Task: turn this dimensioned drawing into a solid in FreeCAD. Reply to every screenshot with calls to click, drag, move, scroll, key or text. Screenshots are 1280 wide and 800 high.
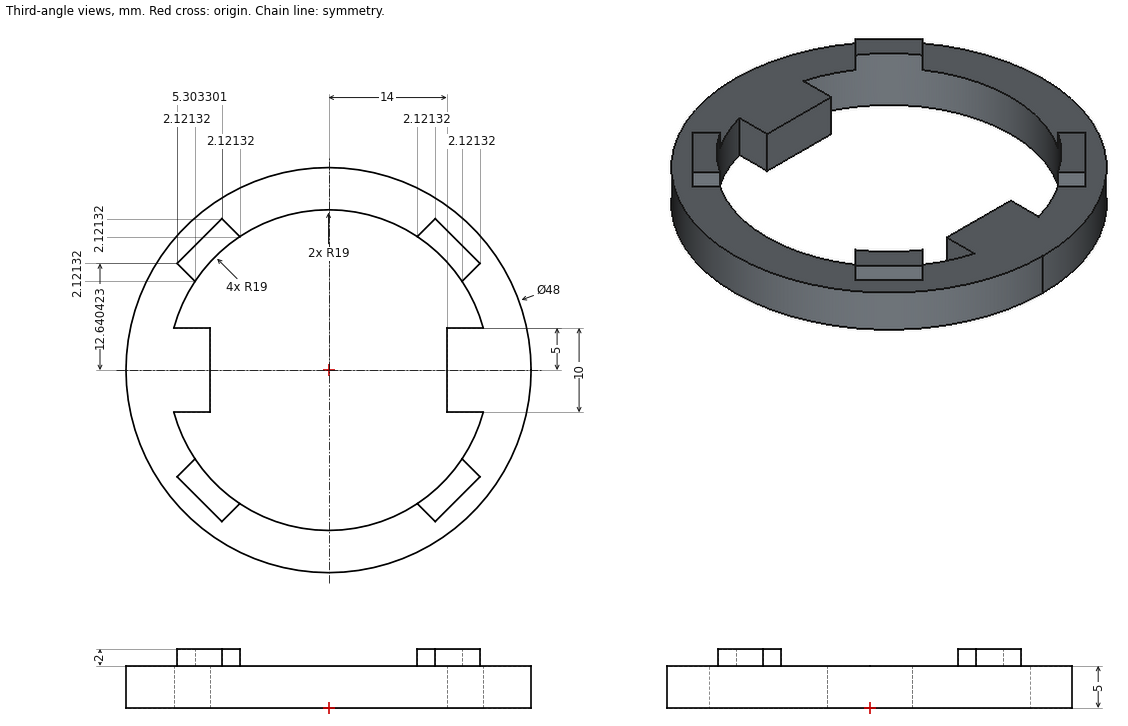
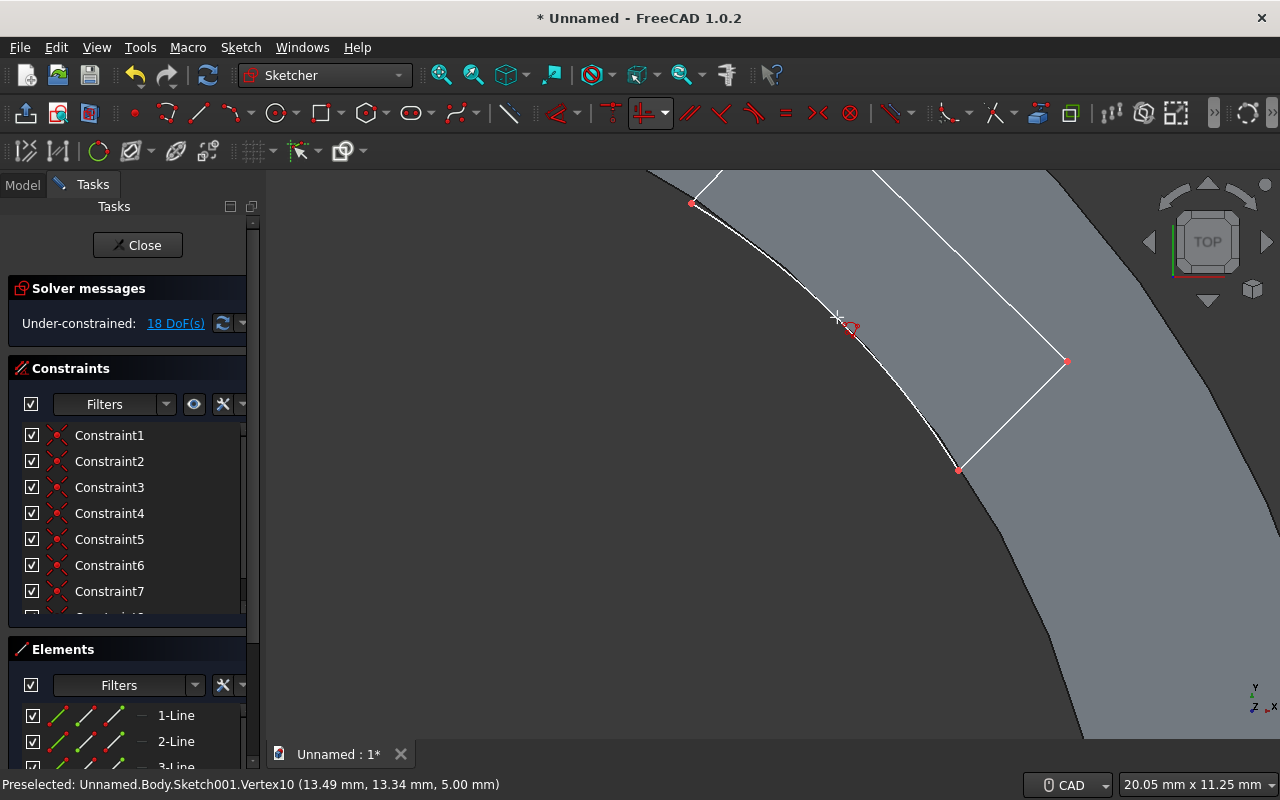
scroll(843, 318, down, 8)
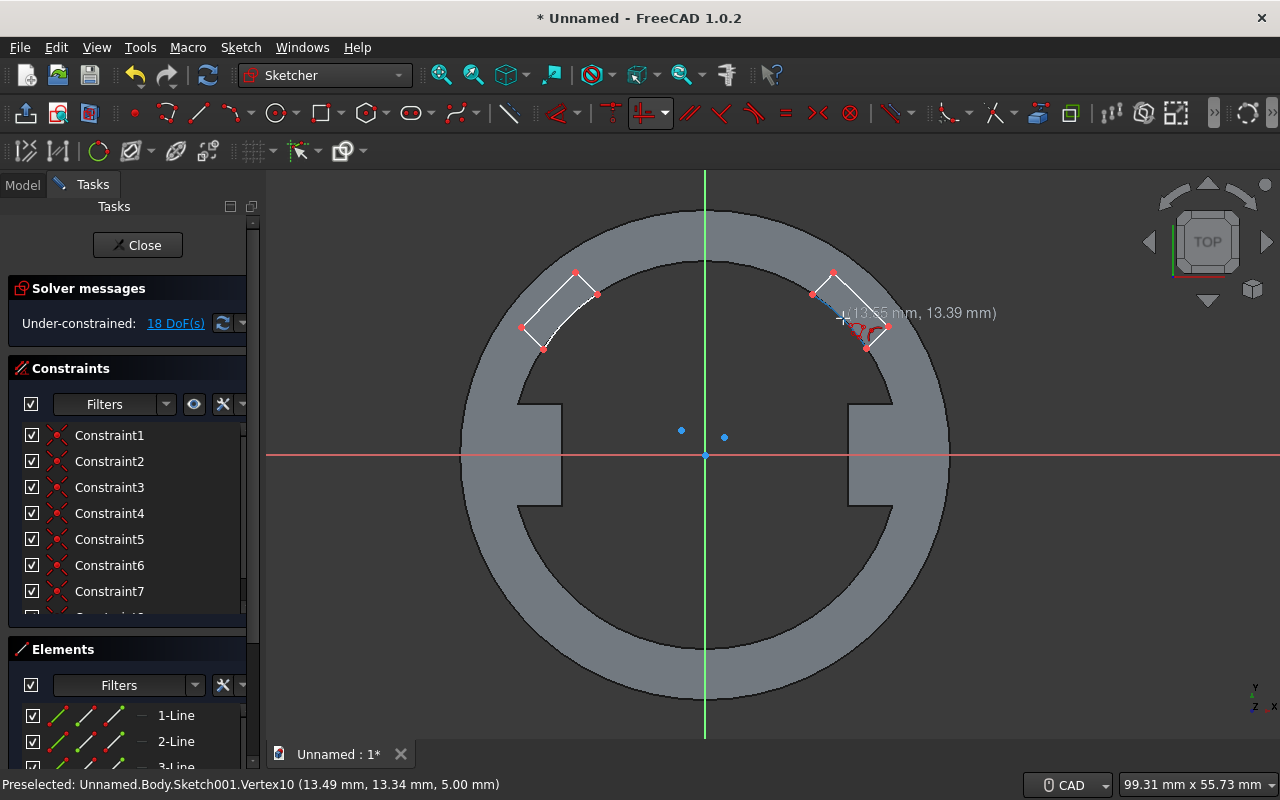
click(813, 617)
click(834, 638)
click(888, 584)
click(867, 562)
right_click(867, 562)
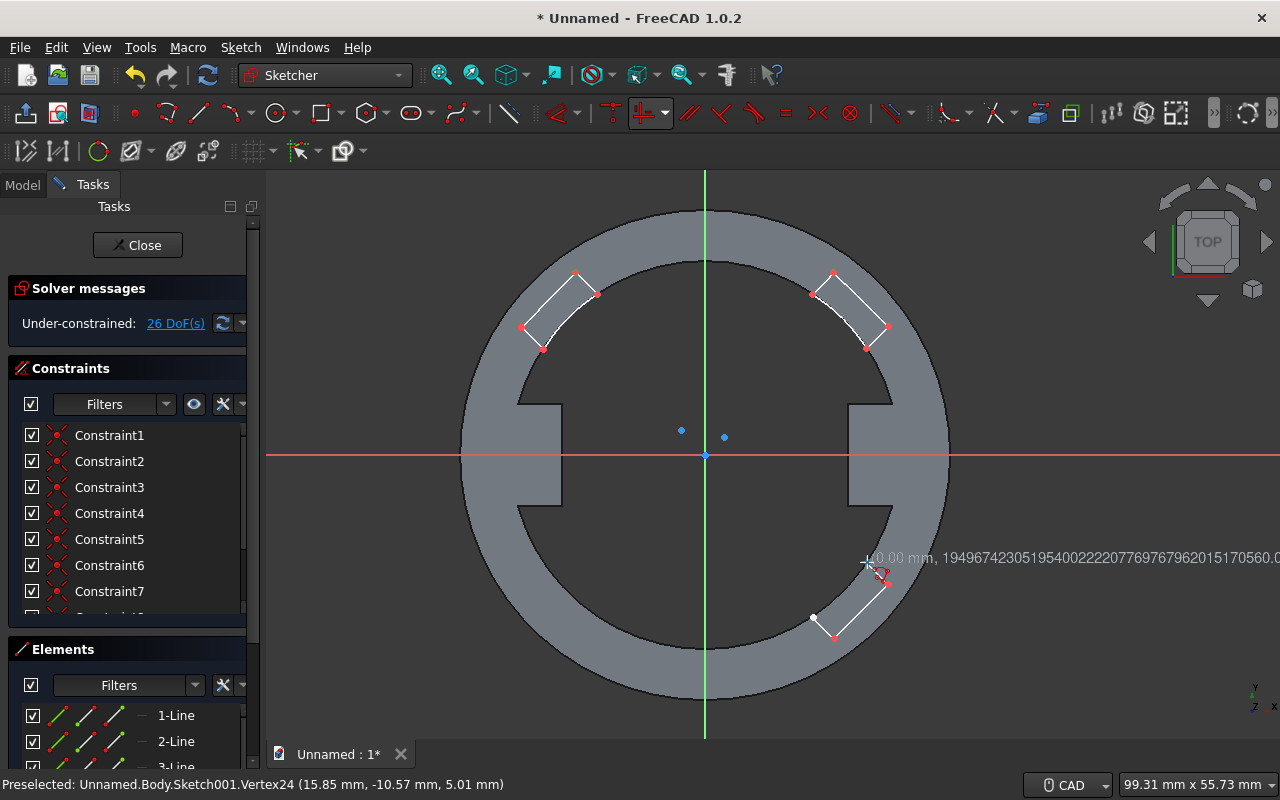
click(232, 114)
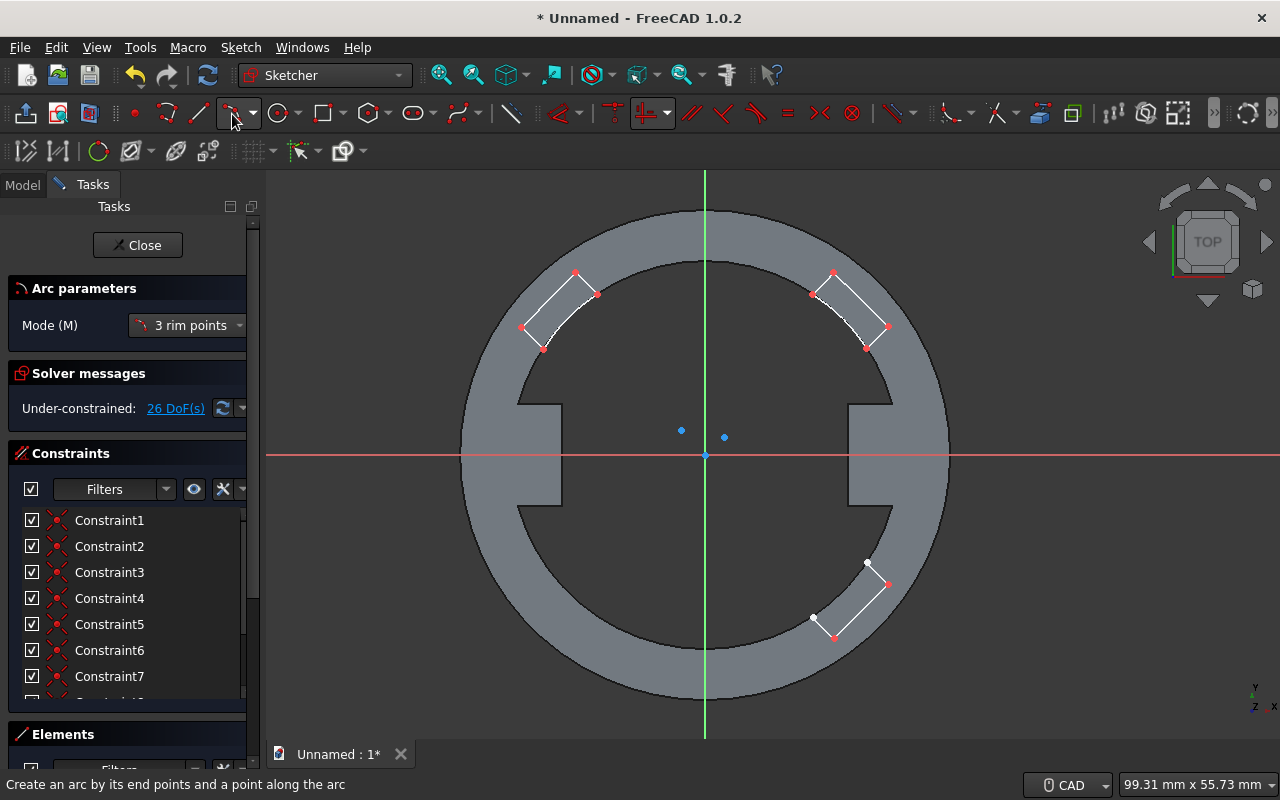
click(867, 563)
click(813, 618)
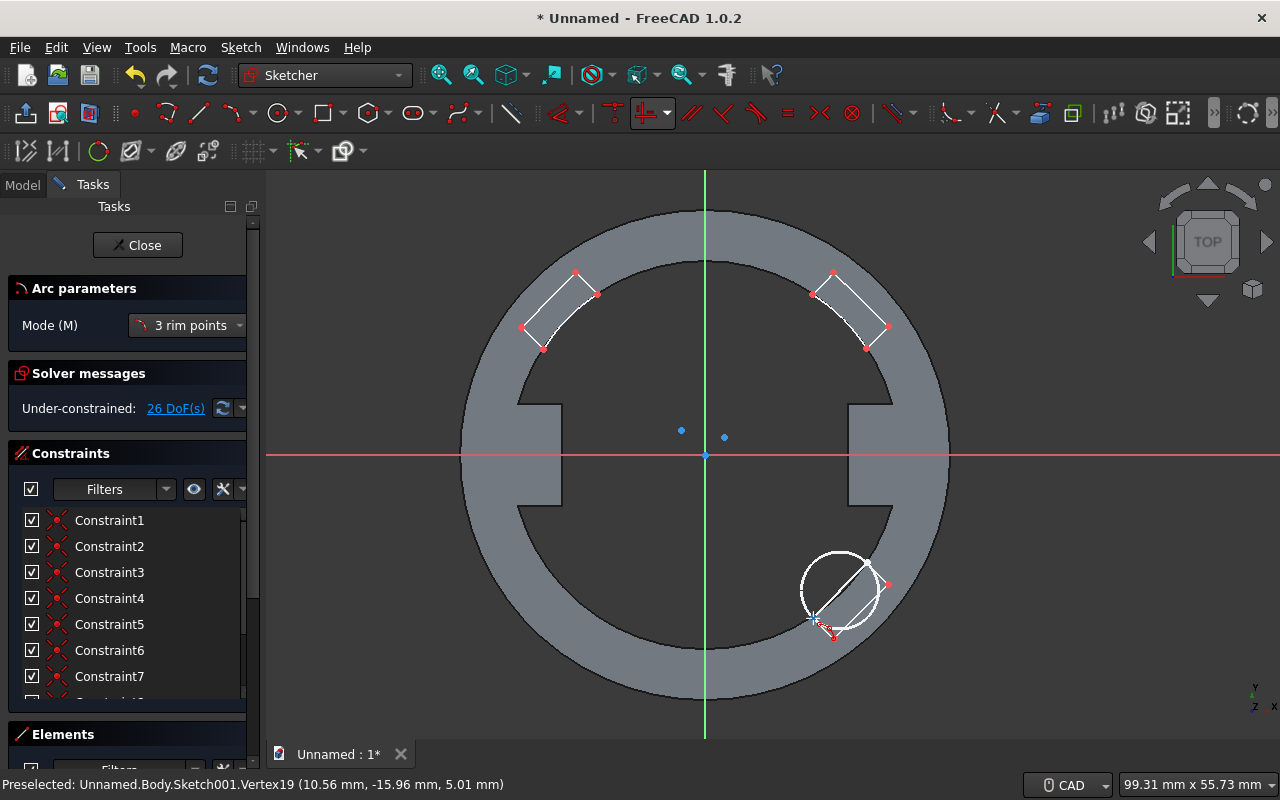
scroll(842, 592, up, 8)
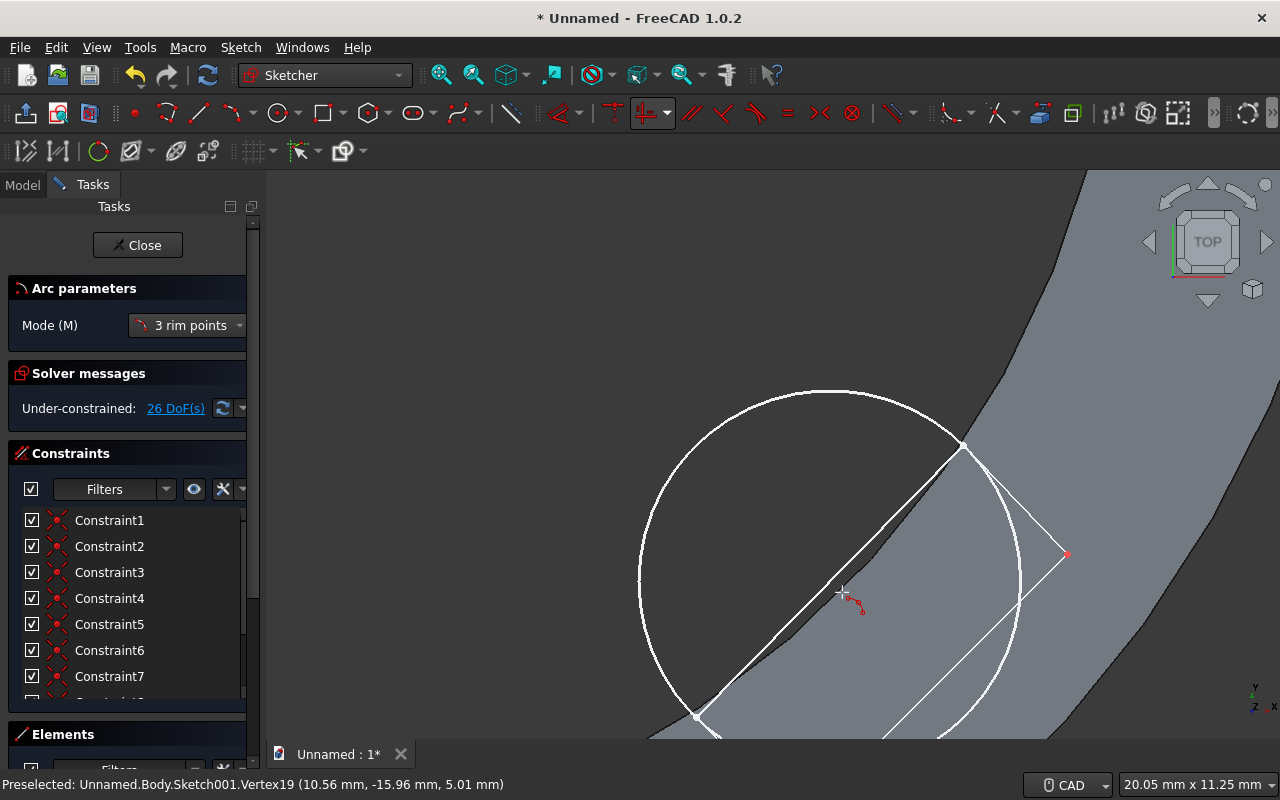
click(841, 590)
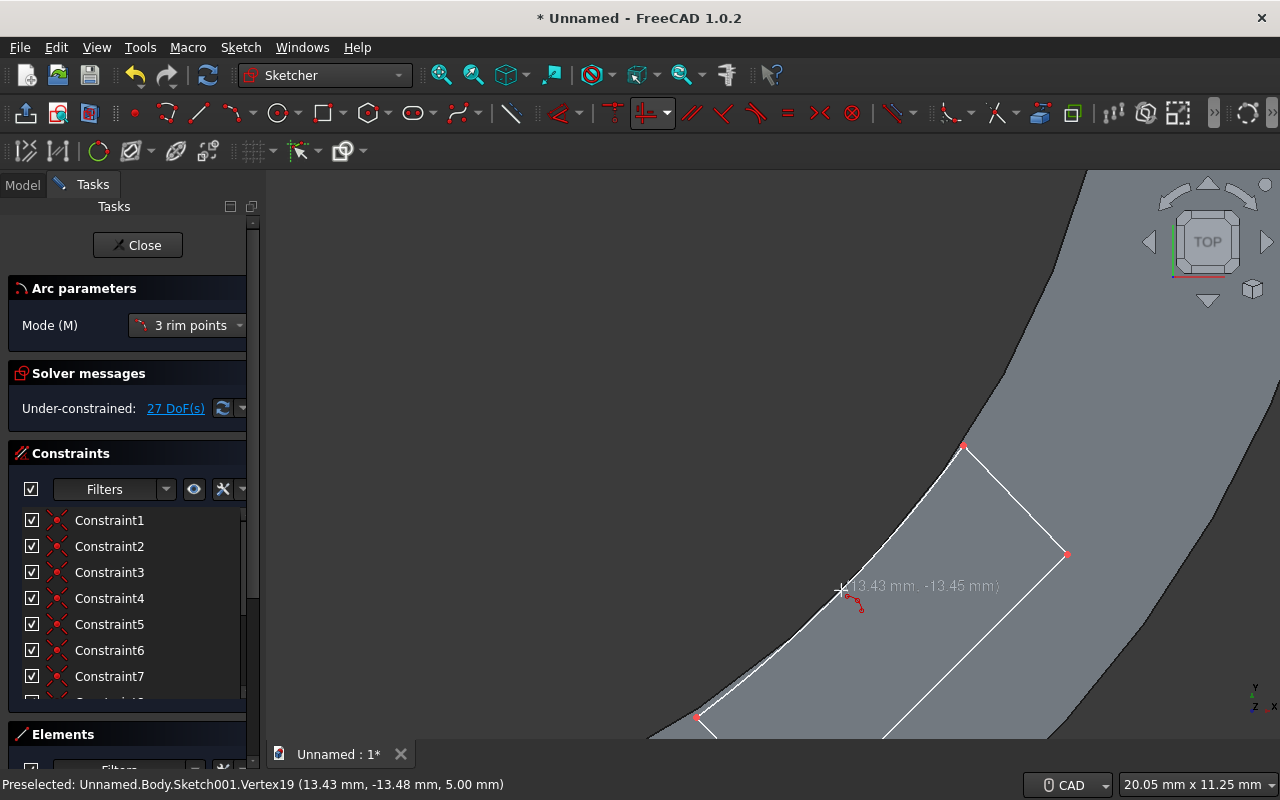
key(g)
key(m)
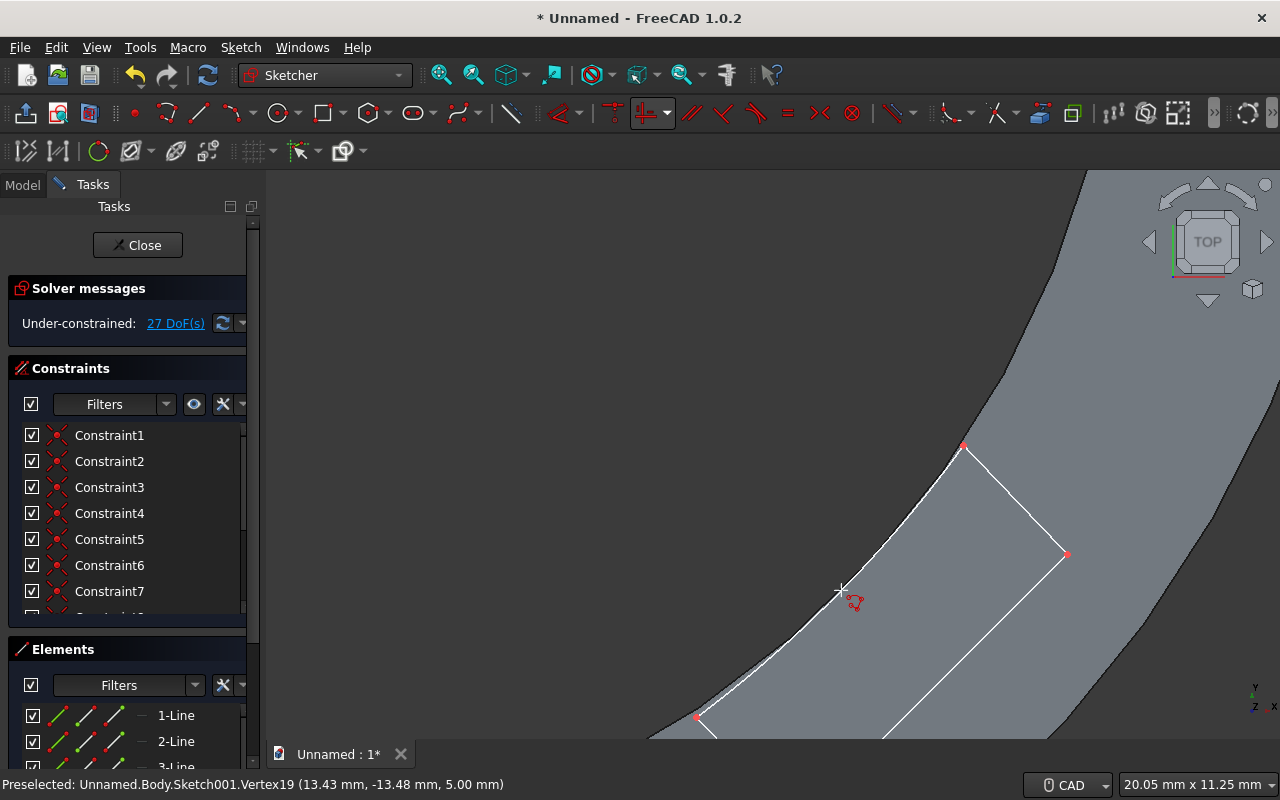
scroll(842, 592, down, 8)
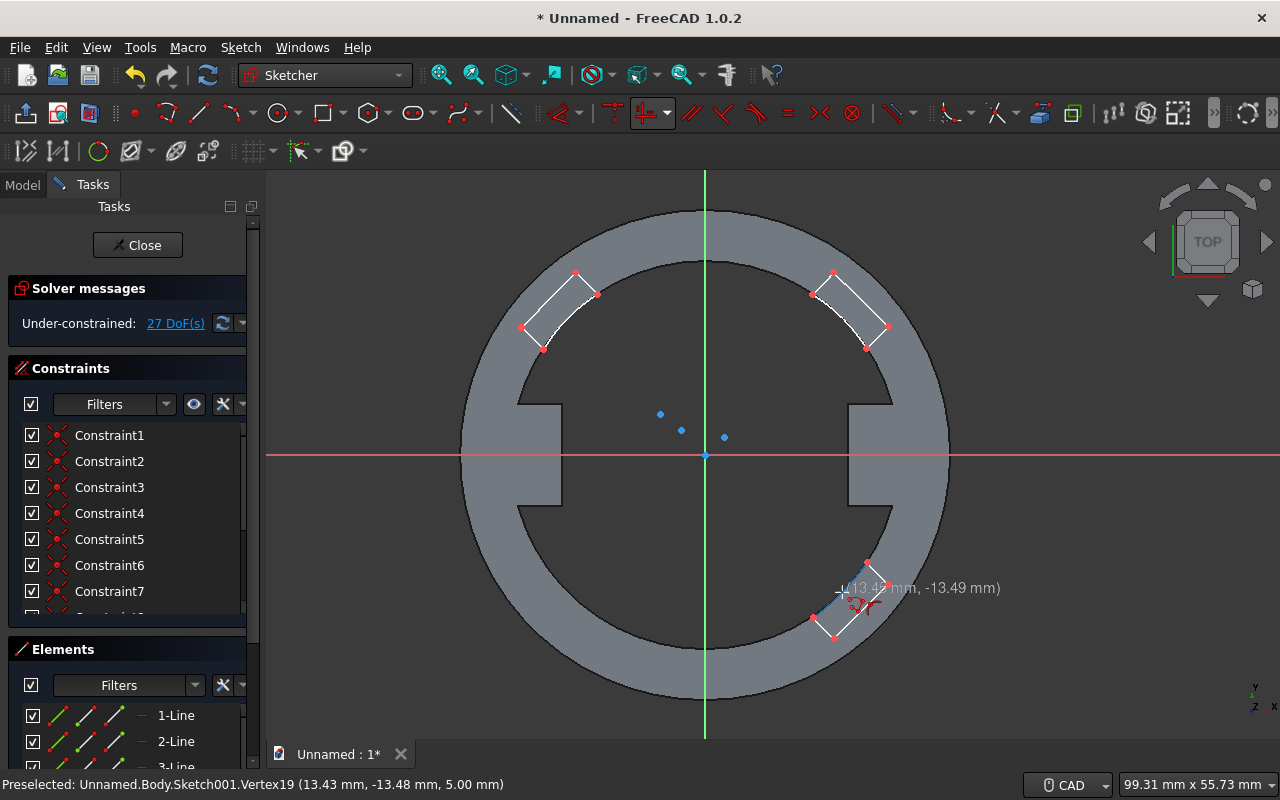
click(544, 562)
click(522, 584)
click(576, 638)
click(598, 617)
right_click(598, 617)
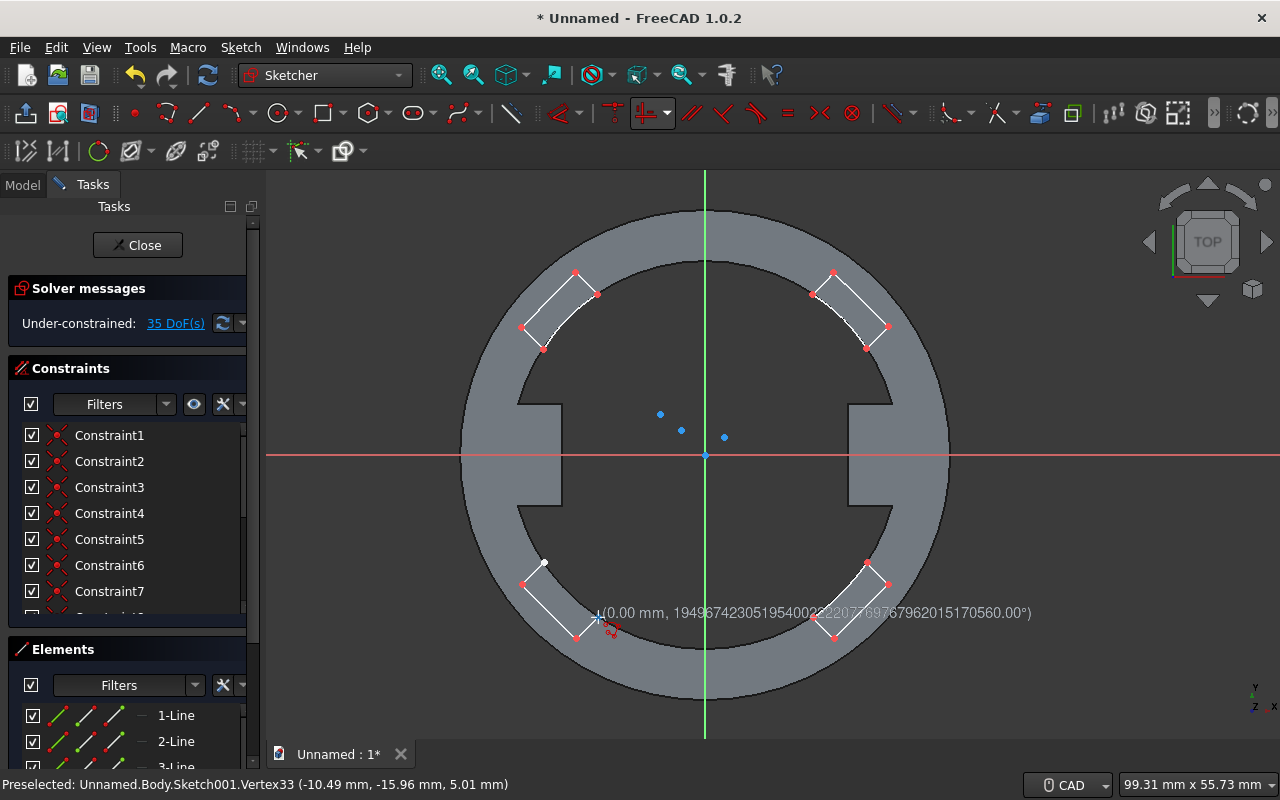
click(232, 114)